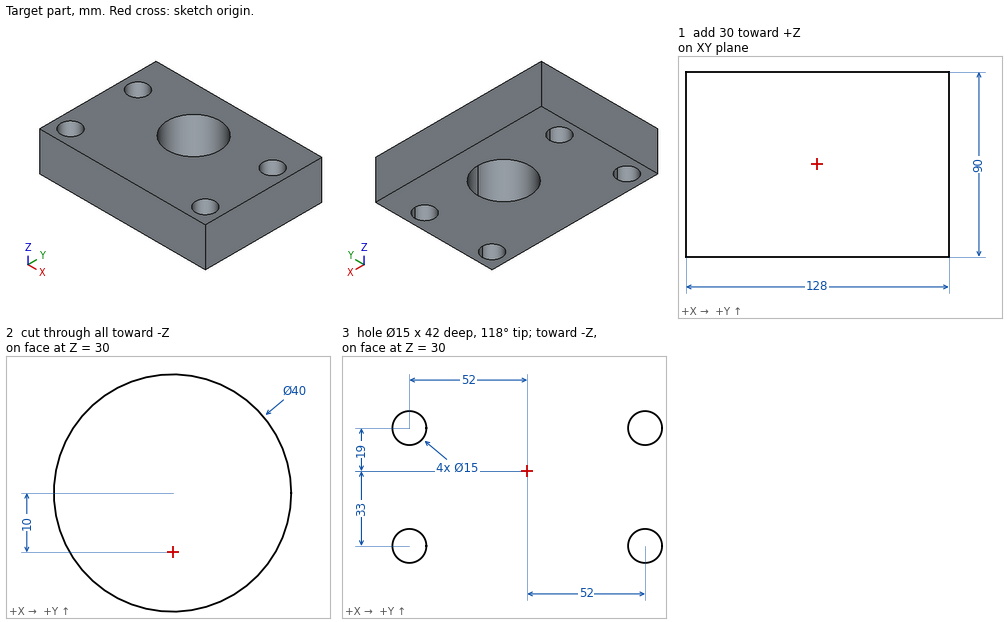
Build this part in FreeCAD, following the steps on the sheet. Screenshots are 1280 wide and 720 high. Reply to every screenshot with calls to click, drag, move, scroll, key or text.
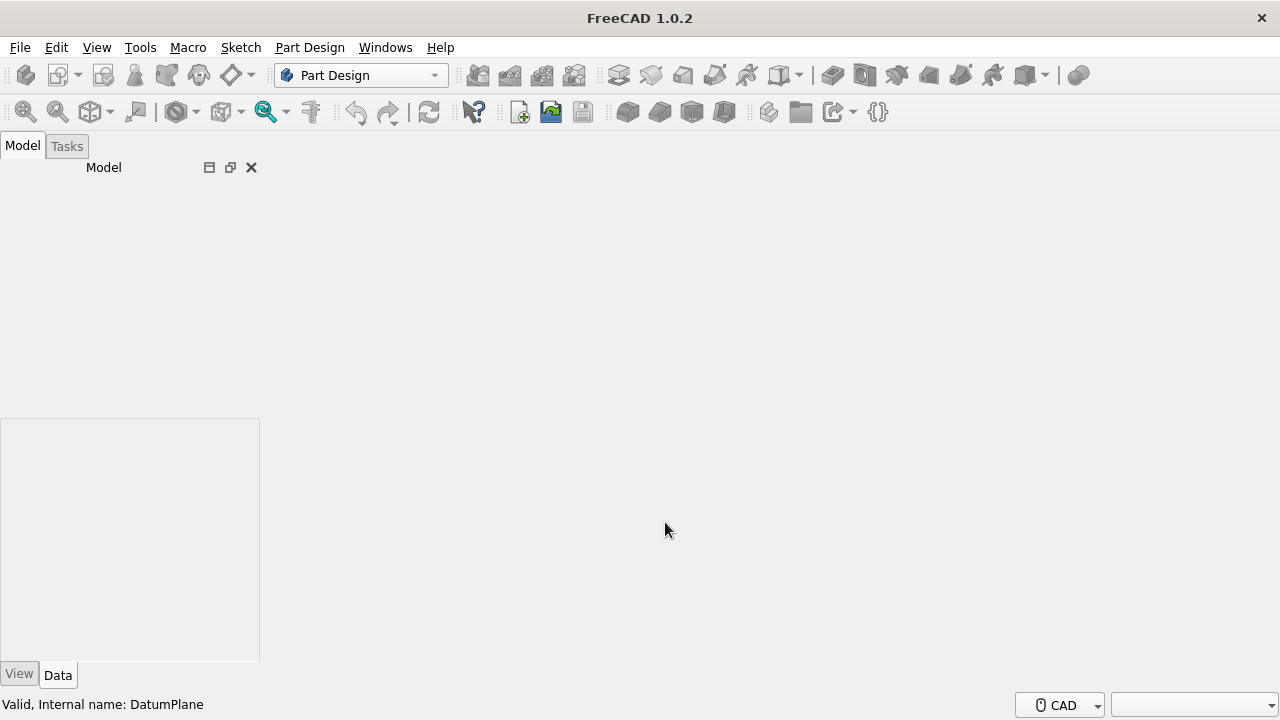
key(ctrl+n)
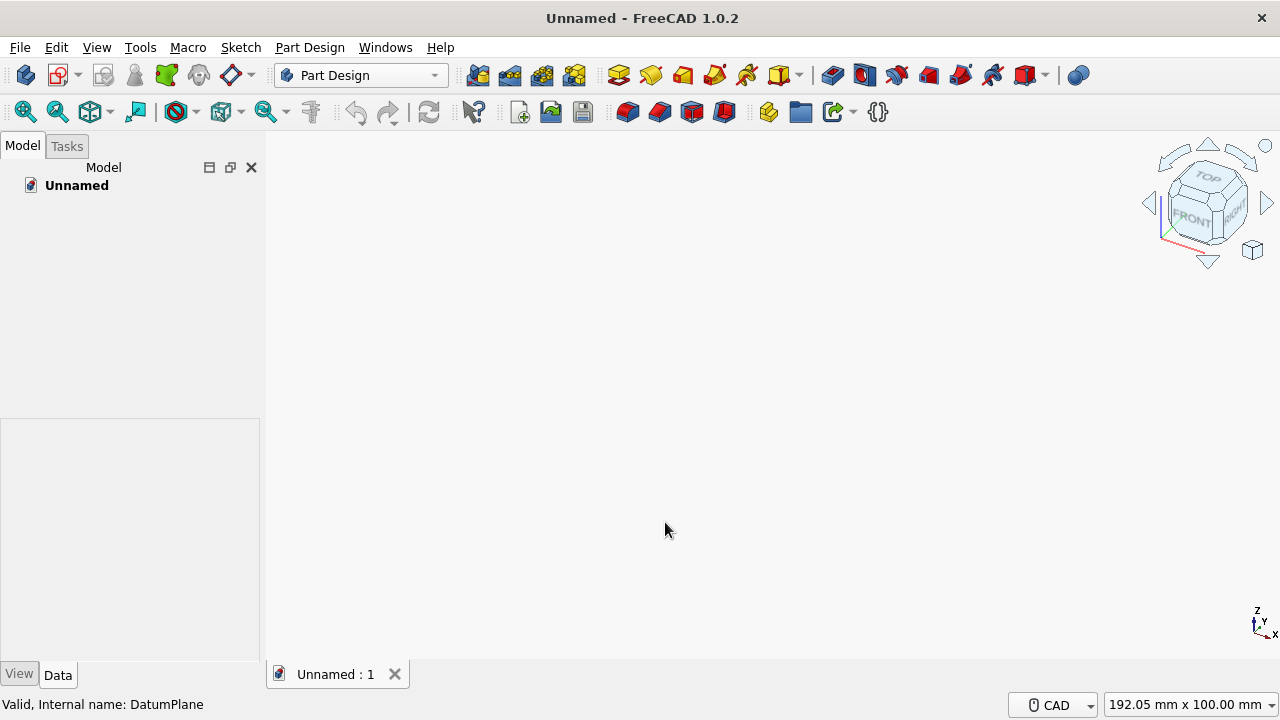
click(58, 76)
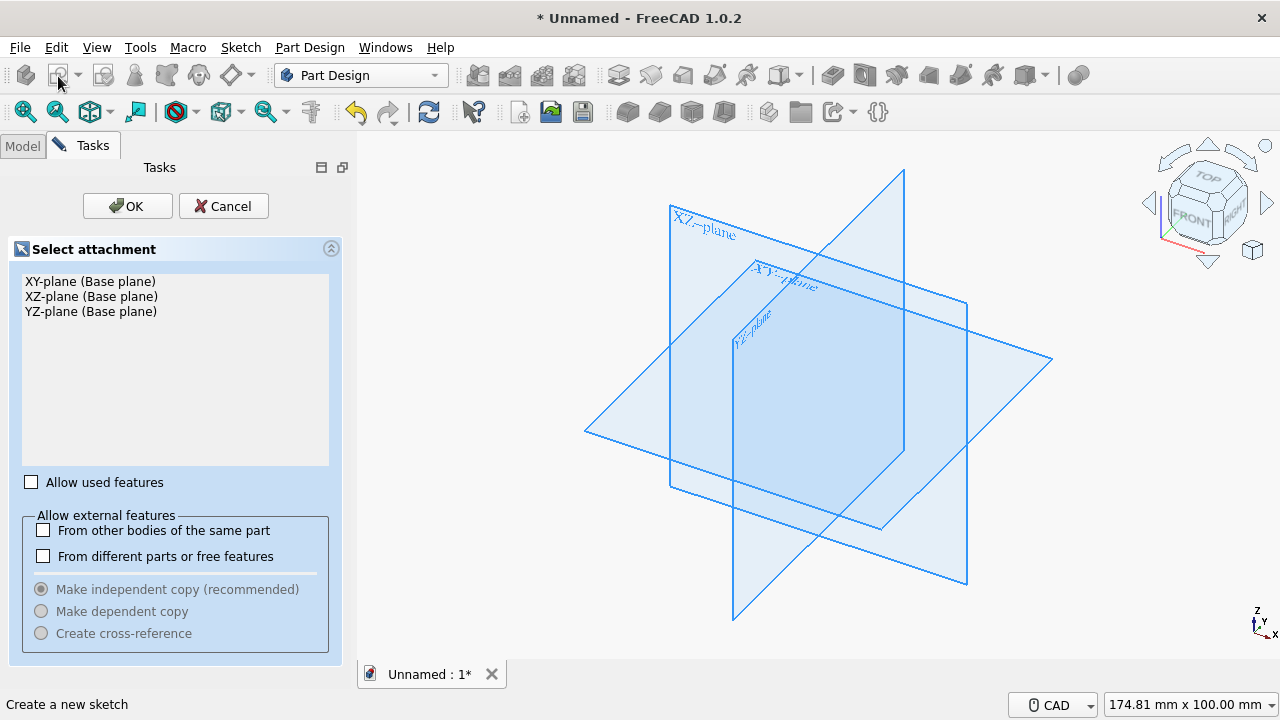
click(82, 282)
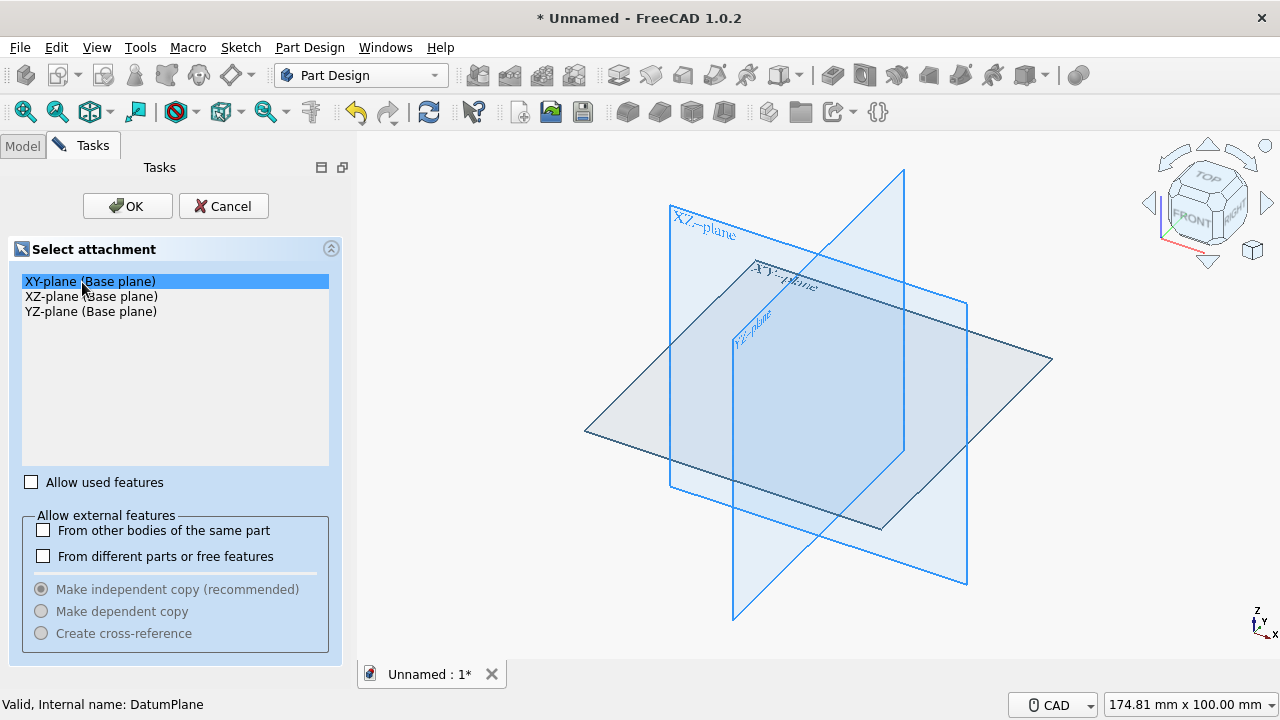
click(128, 206)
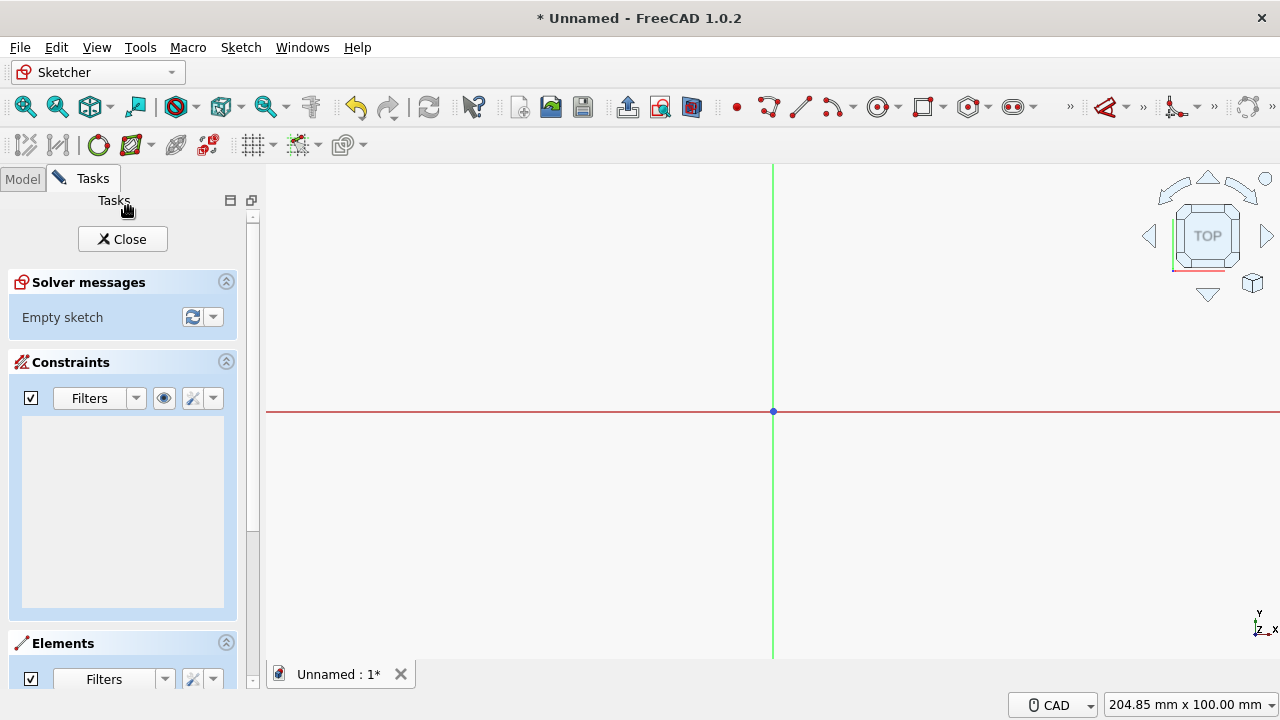
scroll(565, 412, down, 2)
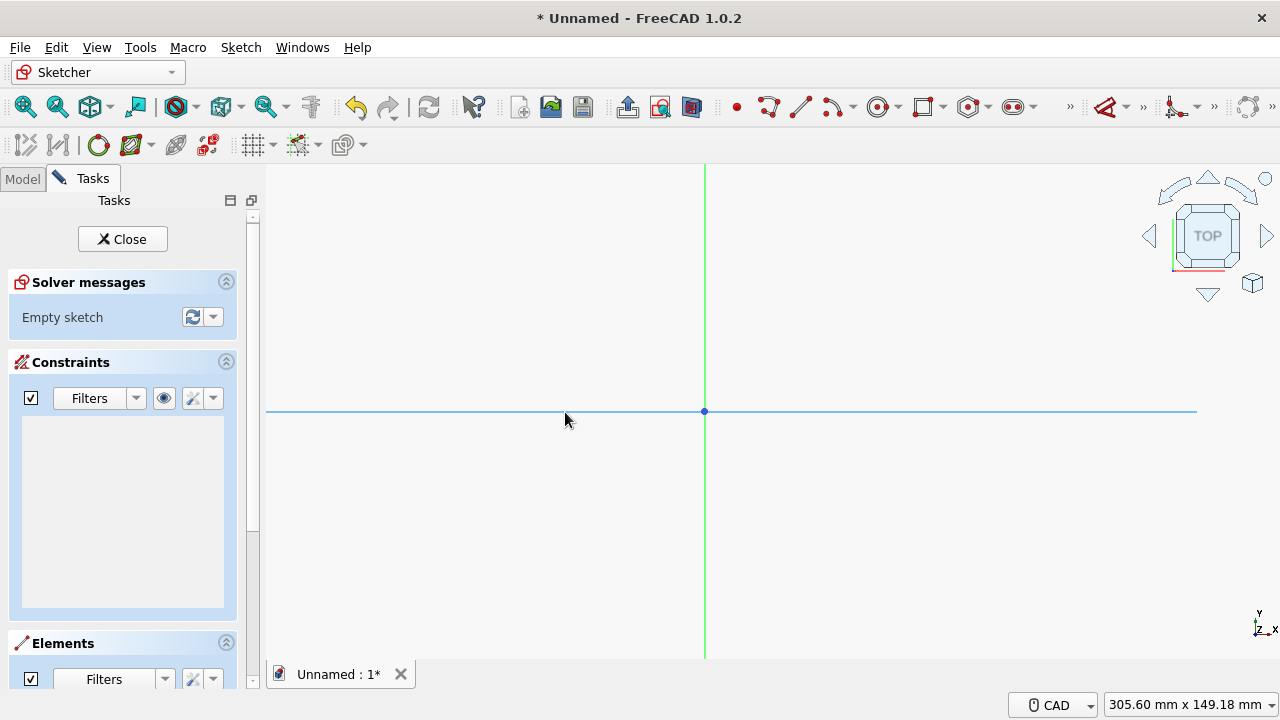
click(946, 108)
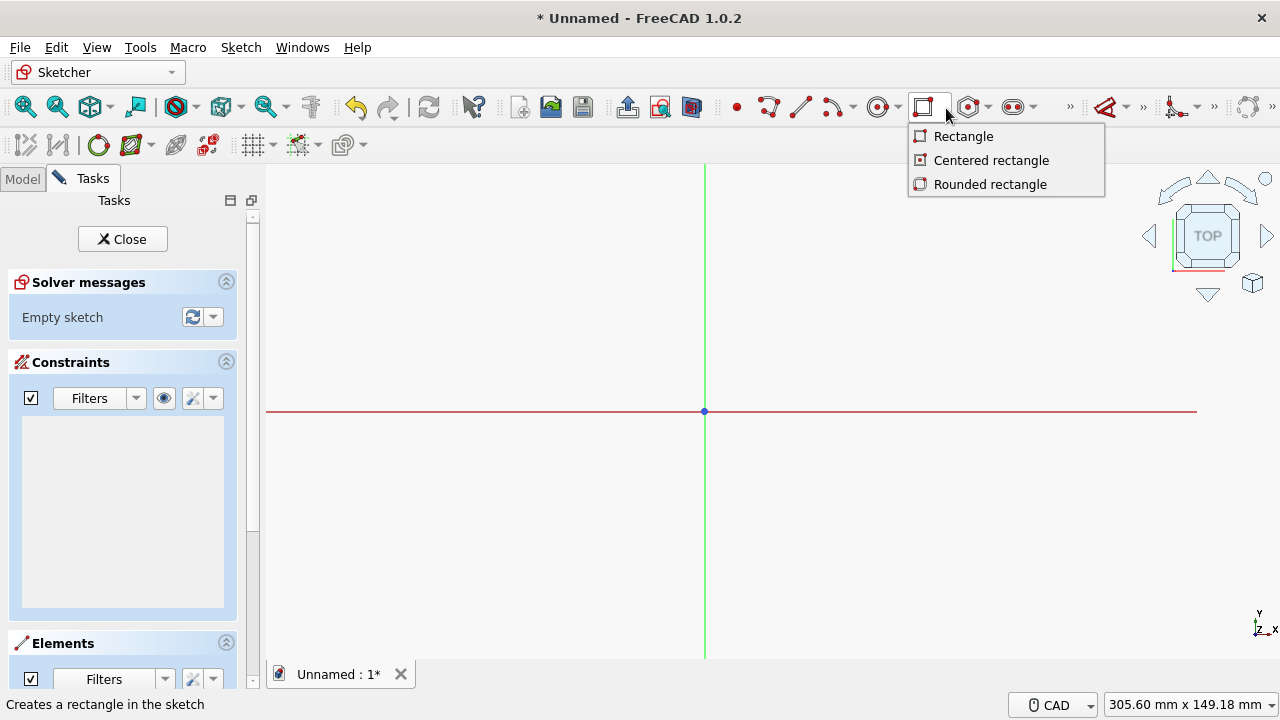
click(1006, 160)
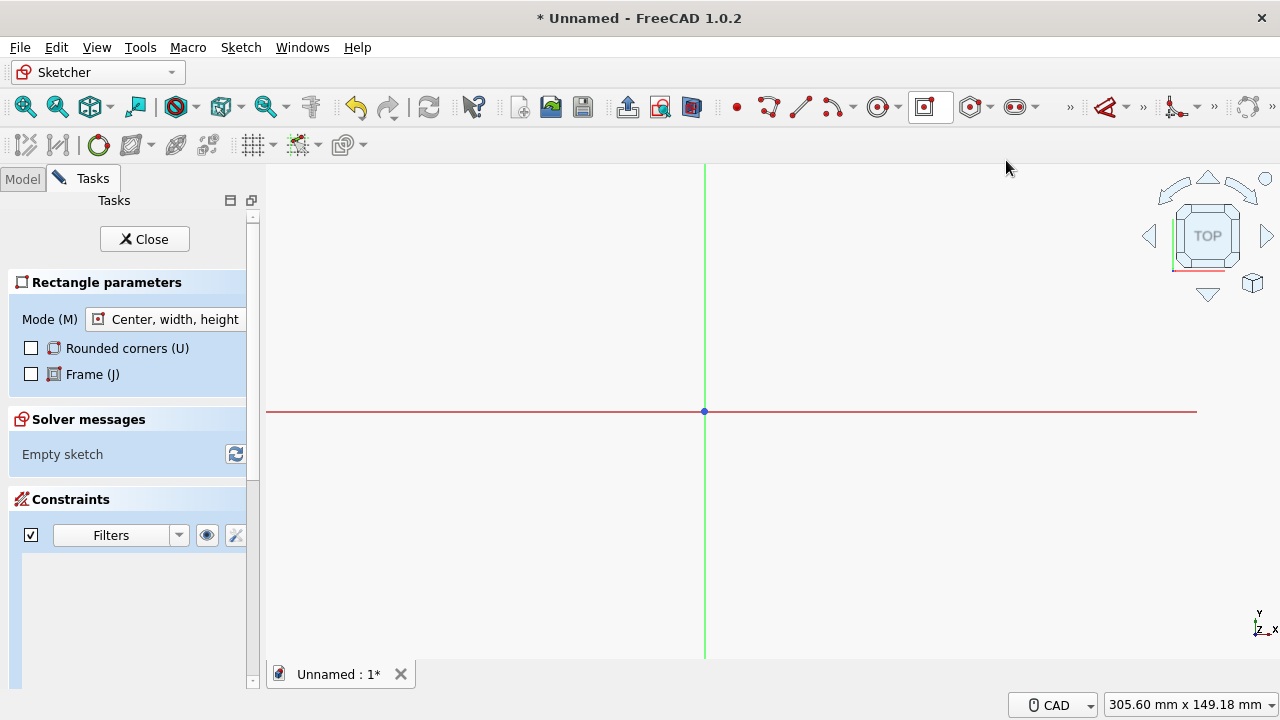
click(705, 412)
click(917, 263)
key(Escape)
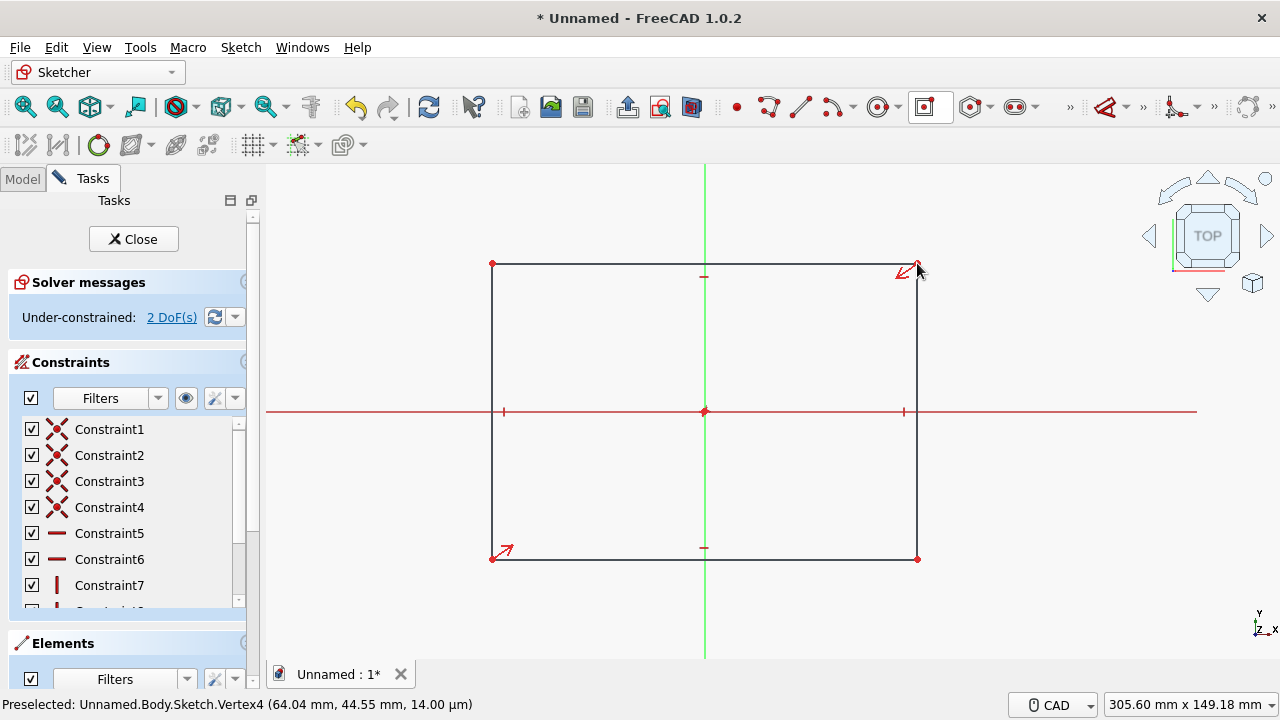
click(917, 471)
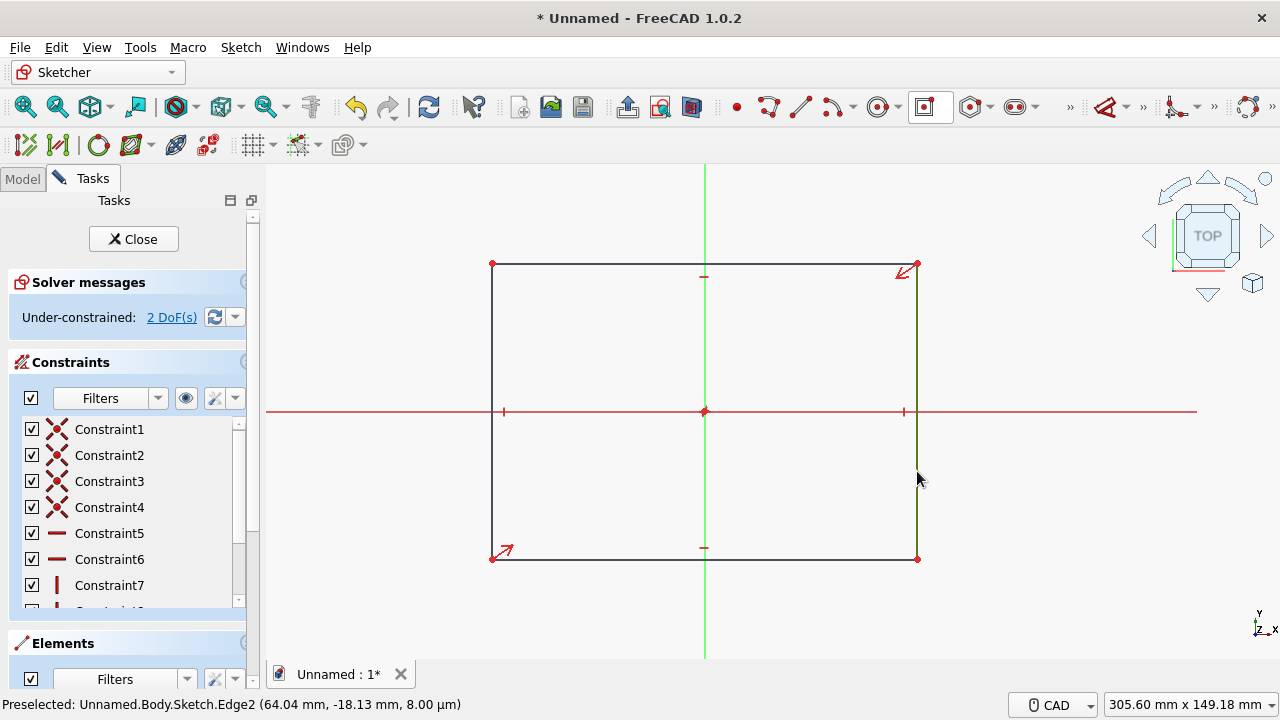
click(1128, 108)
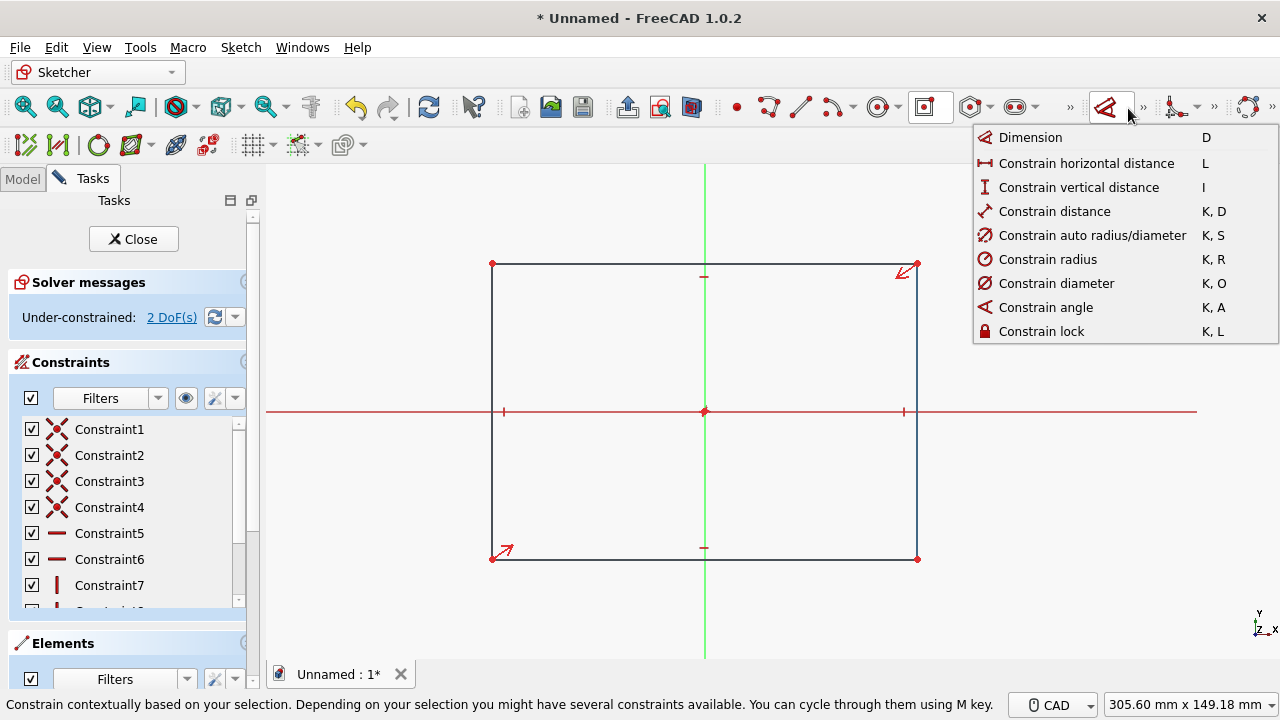
click(1126, 187)